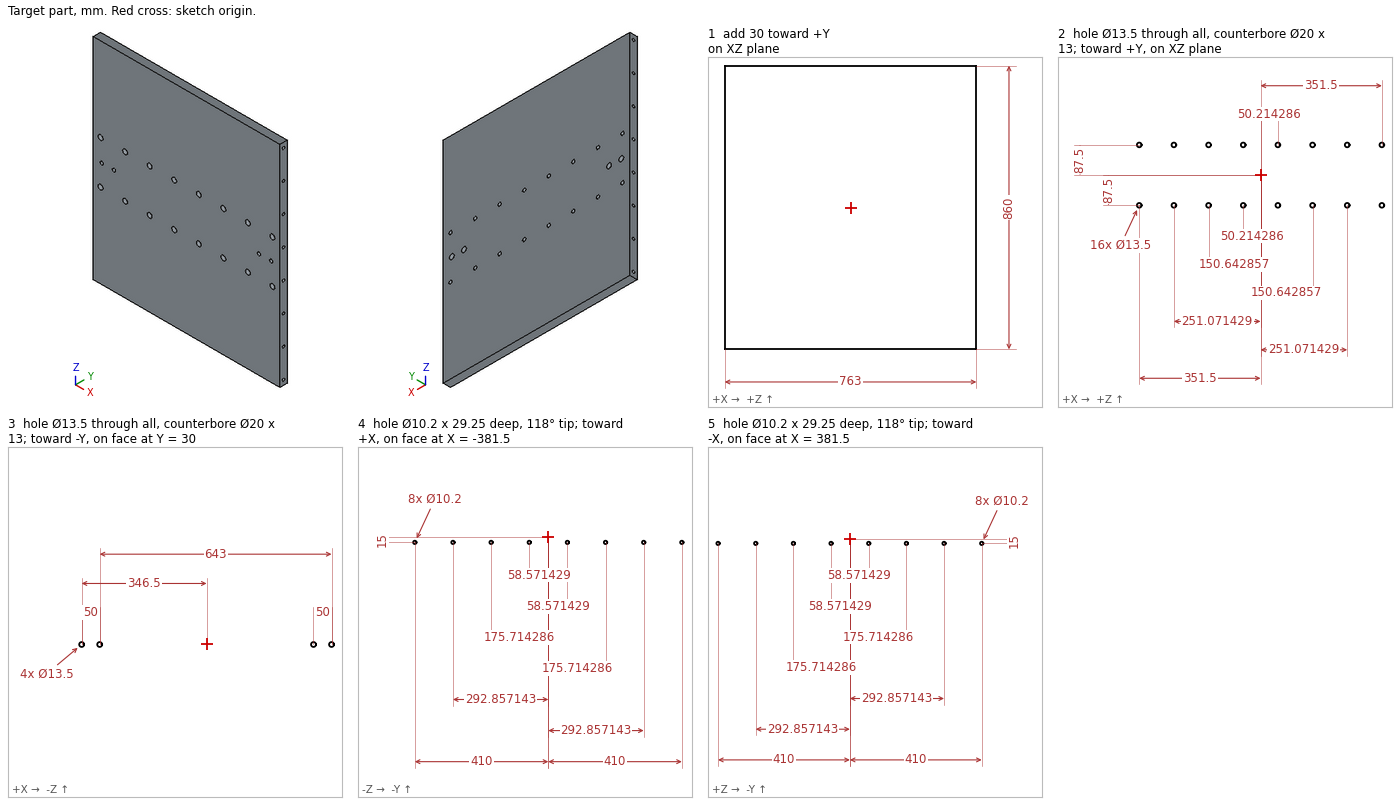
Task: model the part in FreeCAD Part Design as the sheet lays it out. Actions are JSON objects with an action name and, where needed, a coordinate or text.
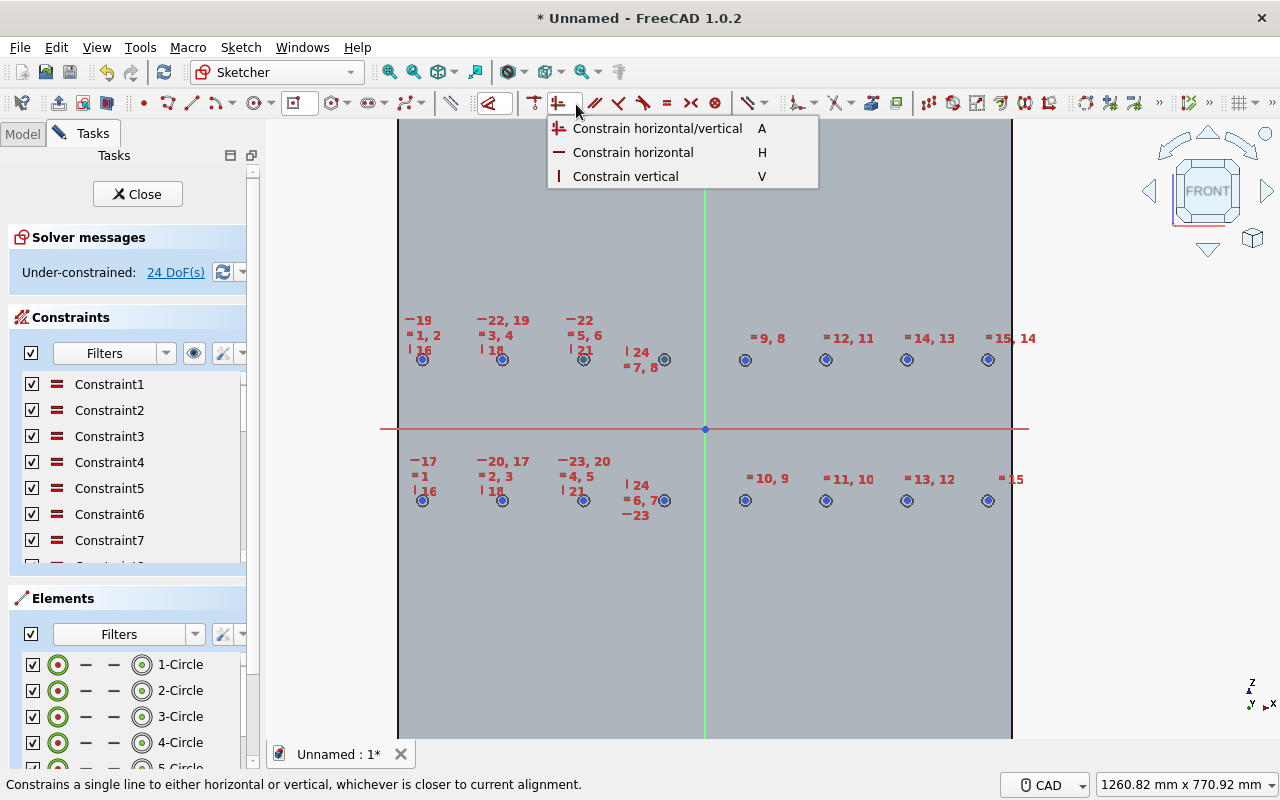
{"action": "left_click", "coordinate": [683, 152]}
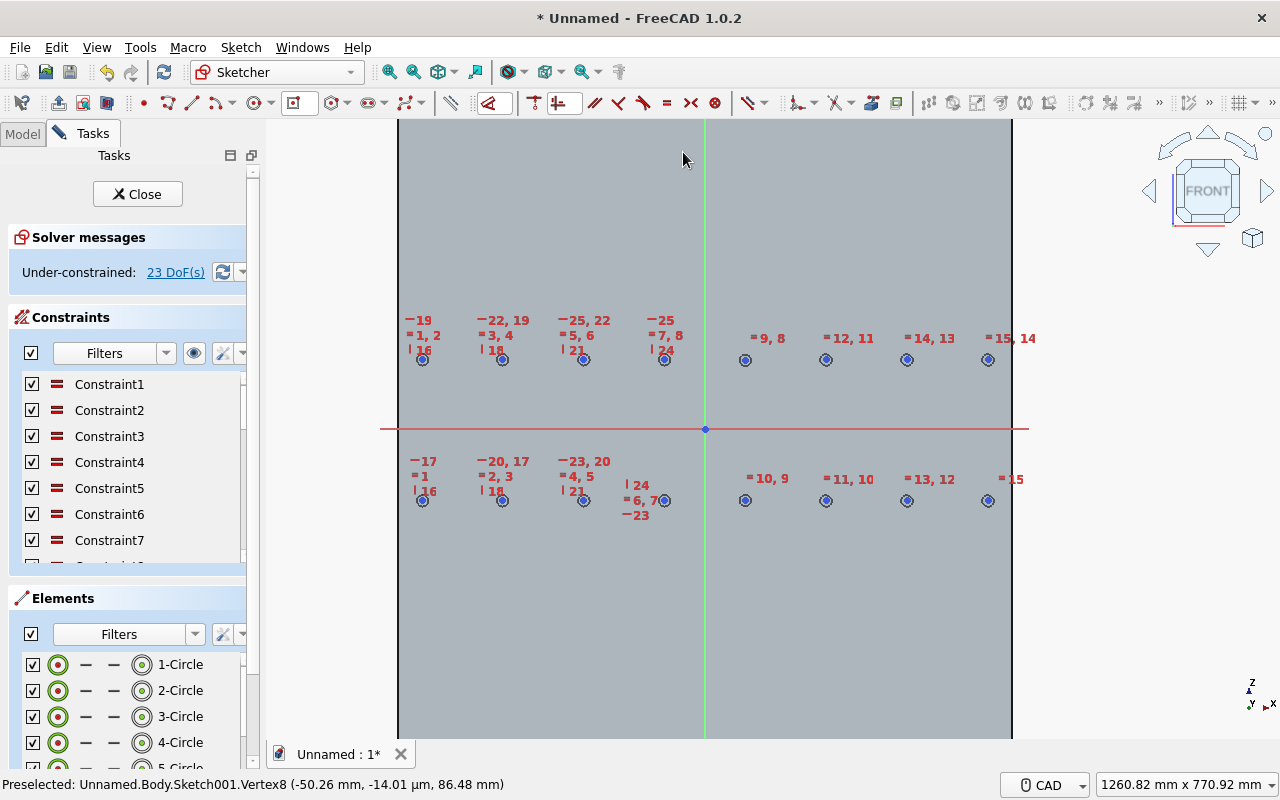
{"action": "left_click", "coordinate": [665, 360]}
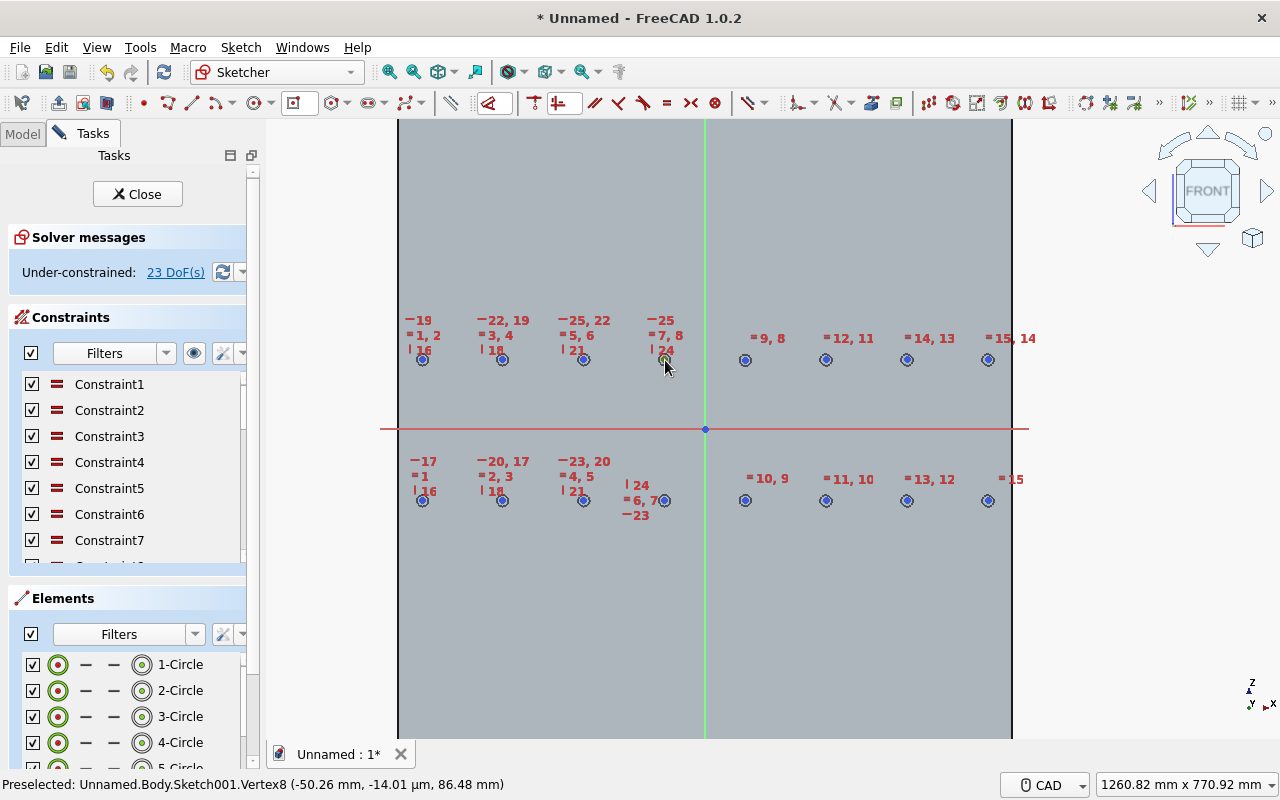
{"action": "left_click", "coordinate": [745, 360]}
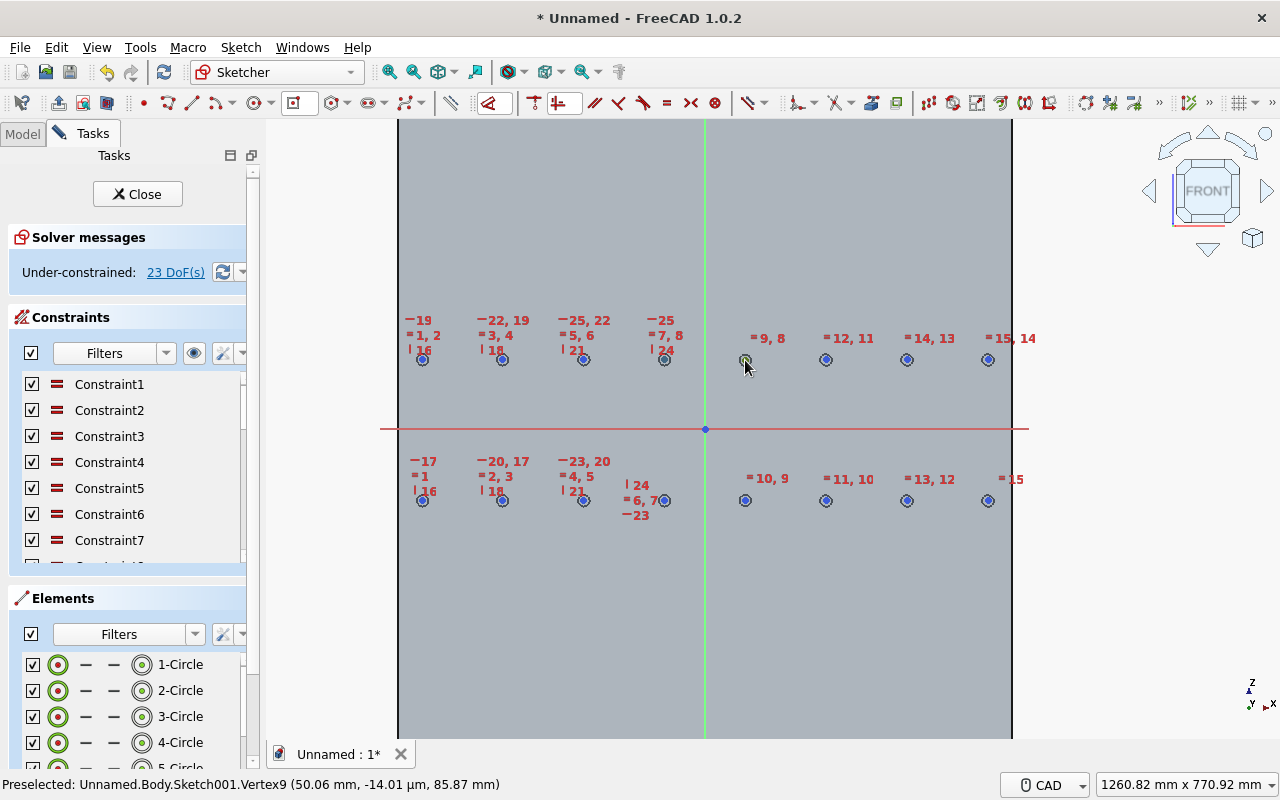
{"action": "key", "text": "h"}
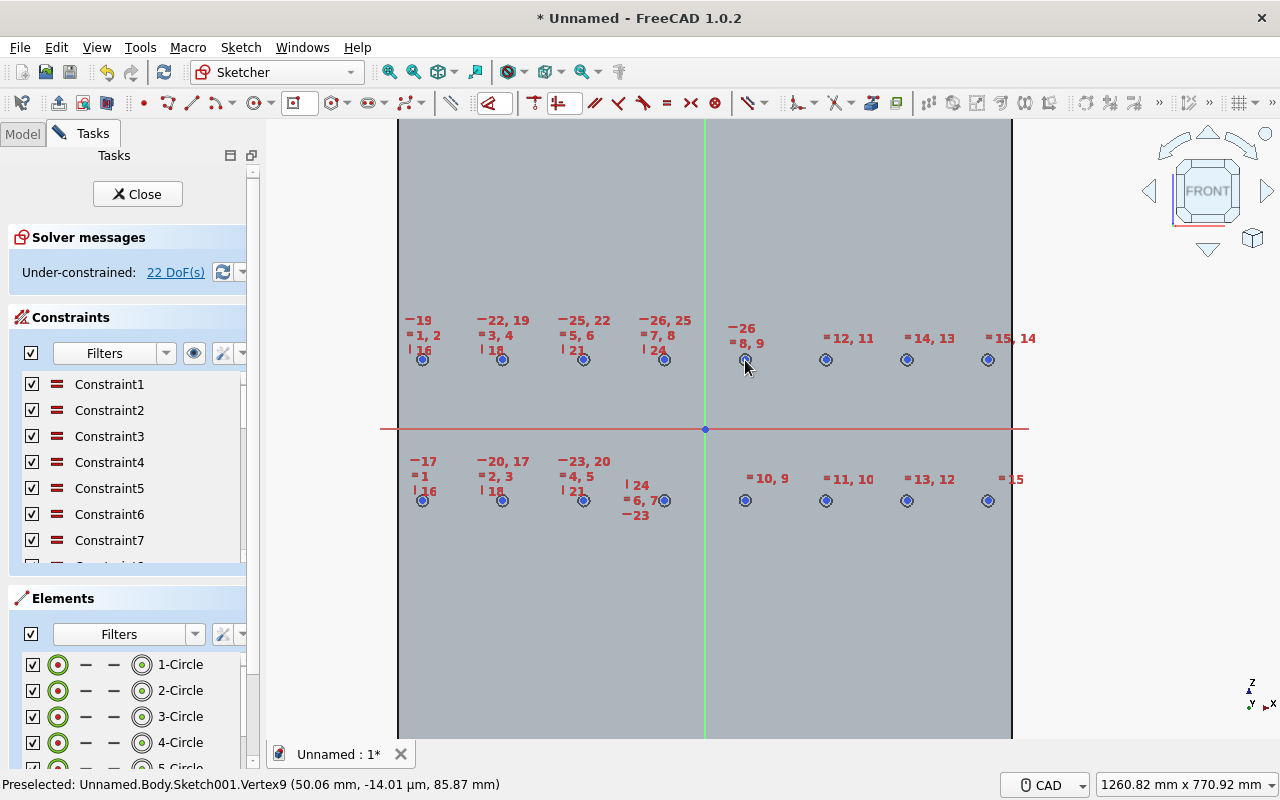
{"action": "left_click", "coordinate": [745, 360]}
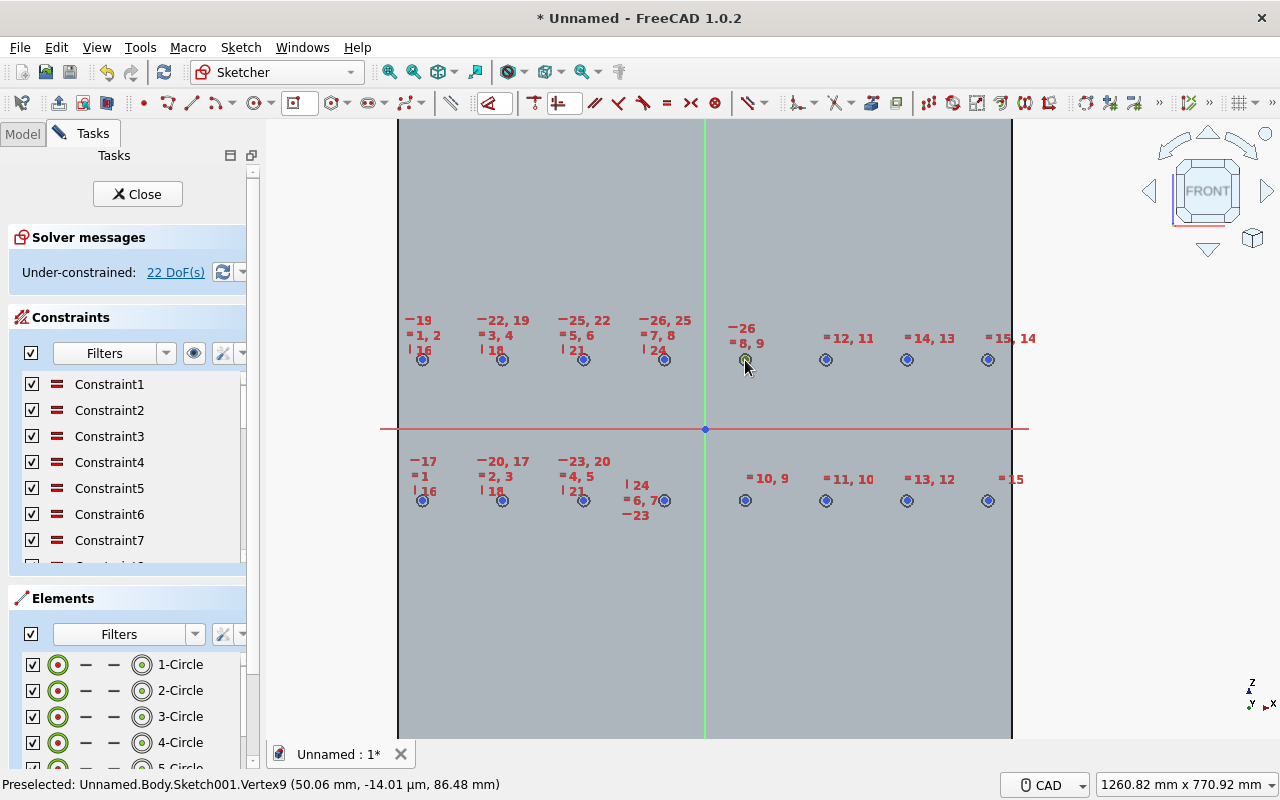
{"action": "left_click", "coordinate": [745, 501]}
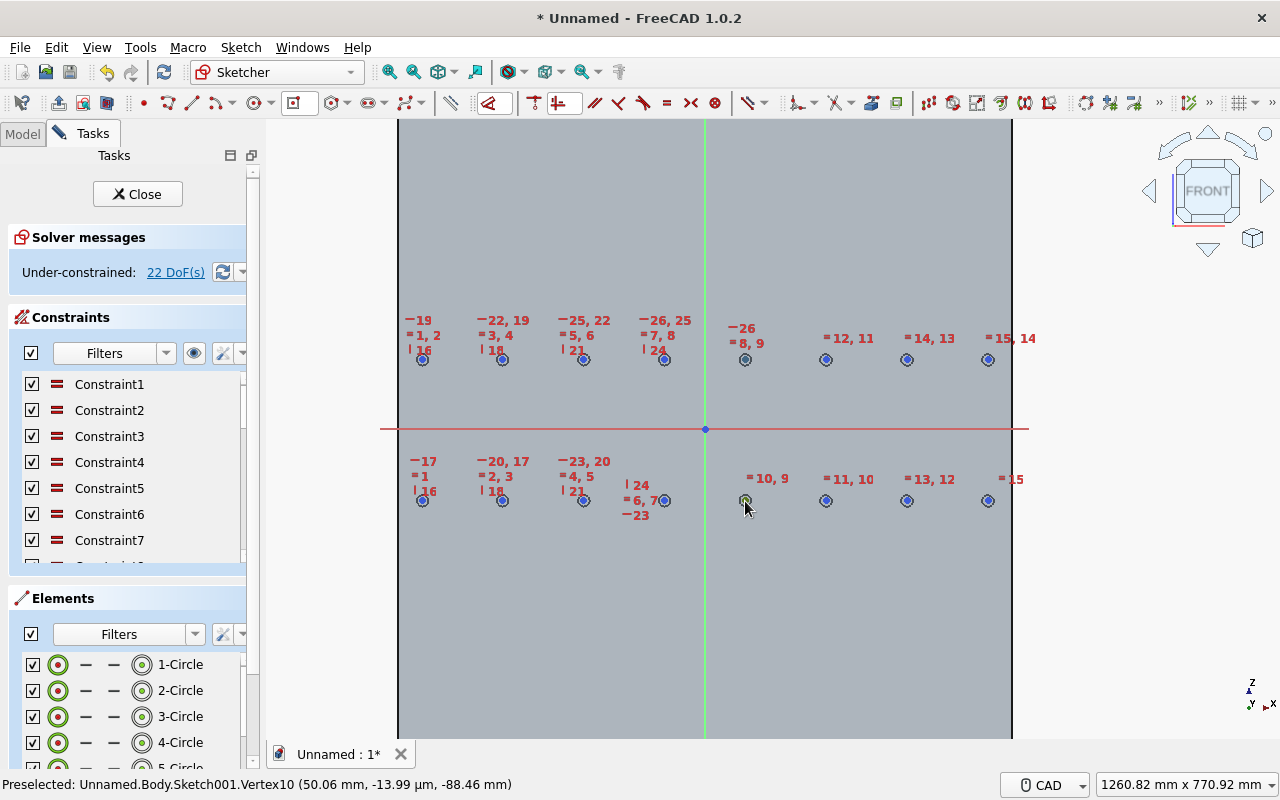
{"action": "left_click", "coordinate": [576, 104]}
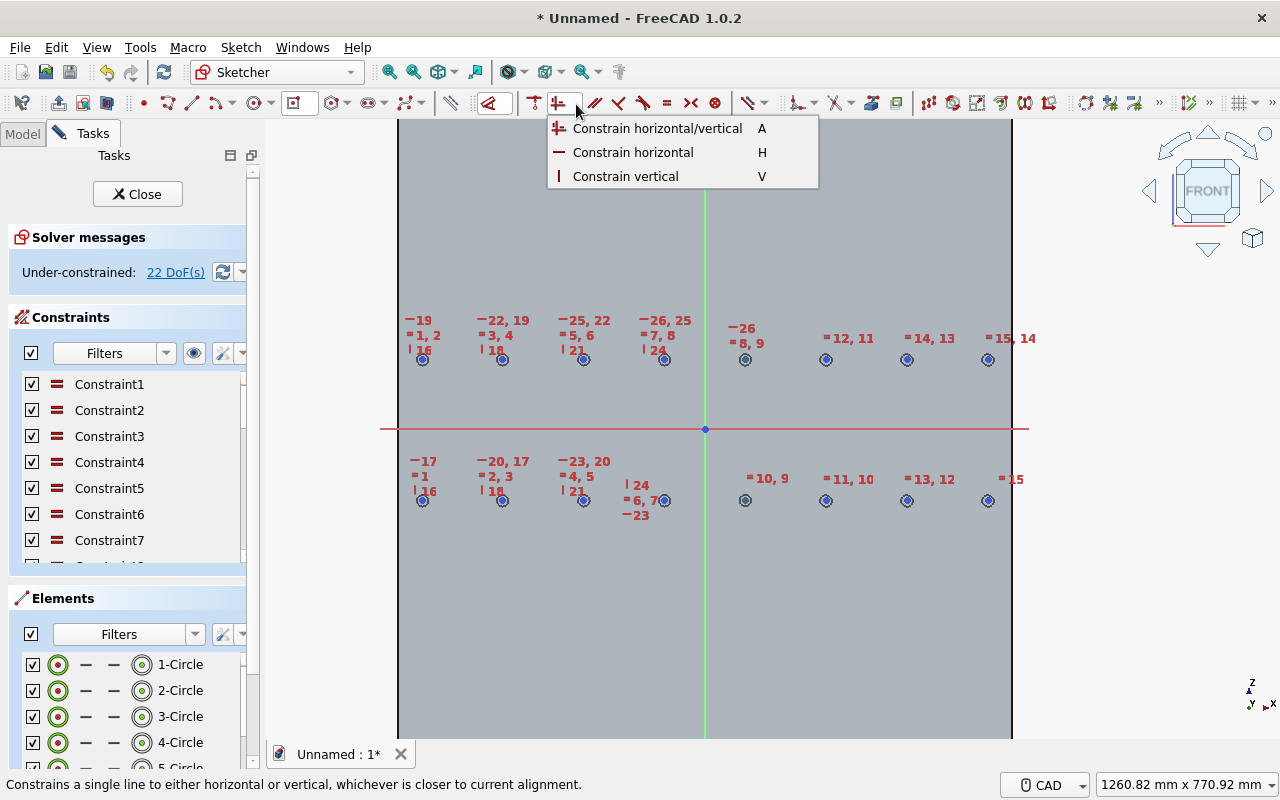
{"action": "left_click", "coordinate": [683, 176]}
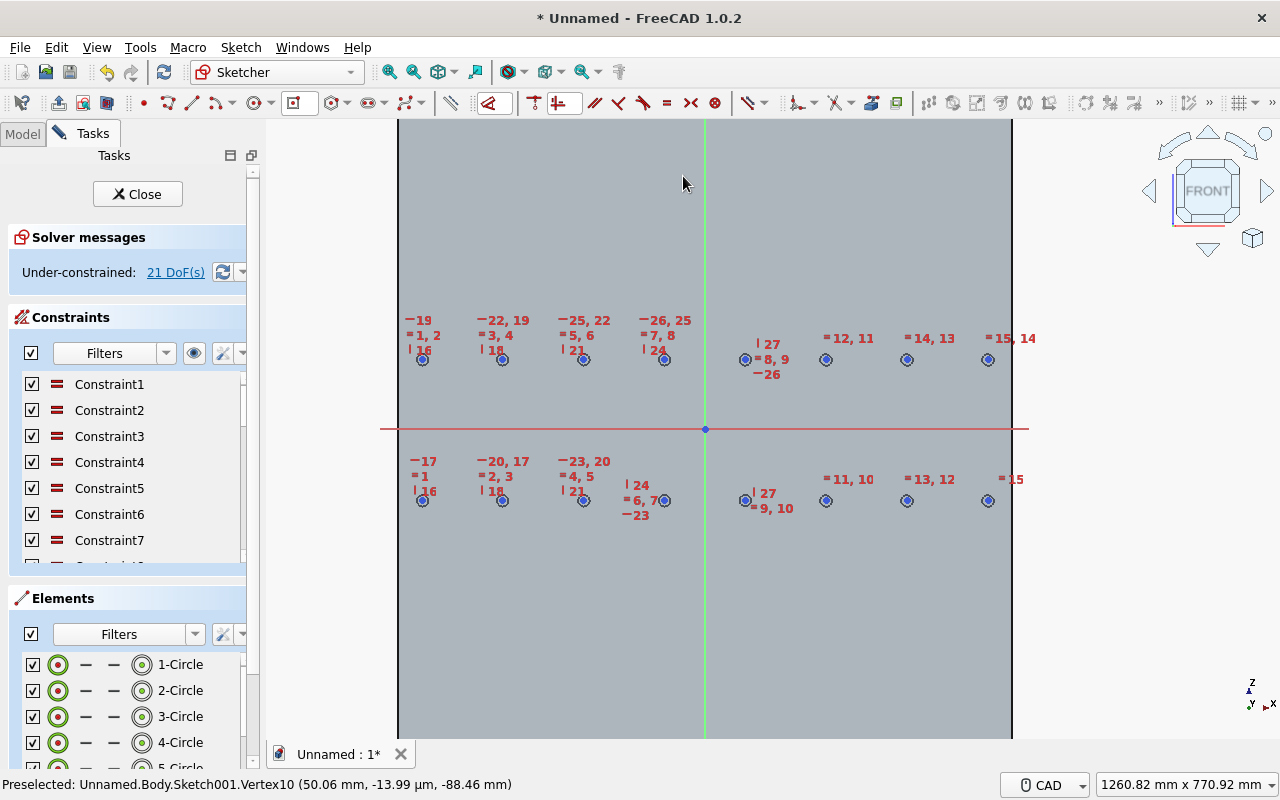
{"action": "left_click", "coordinate": [665, 501]}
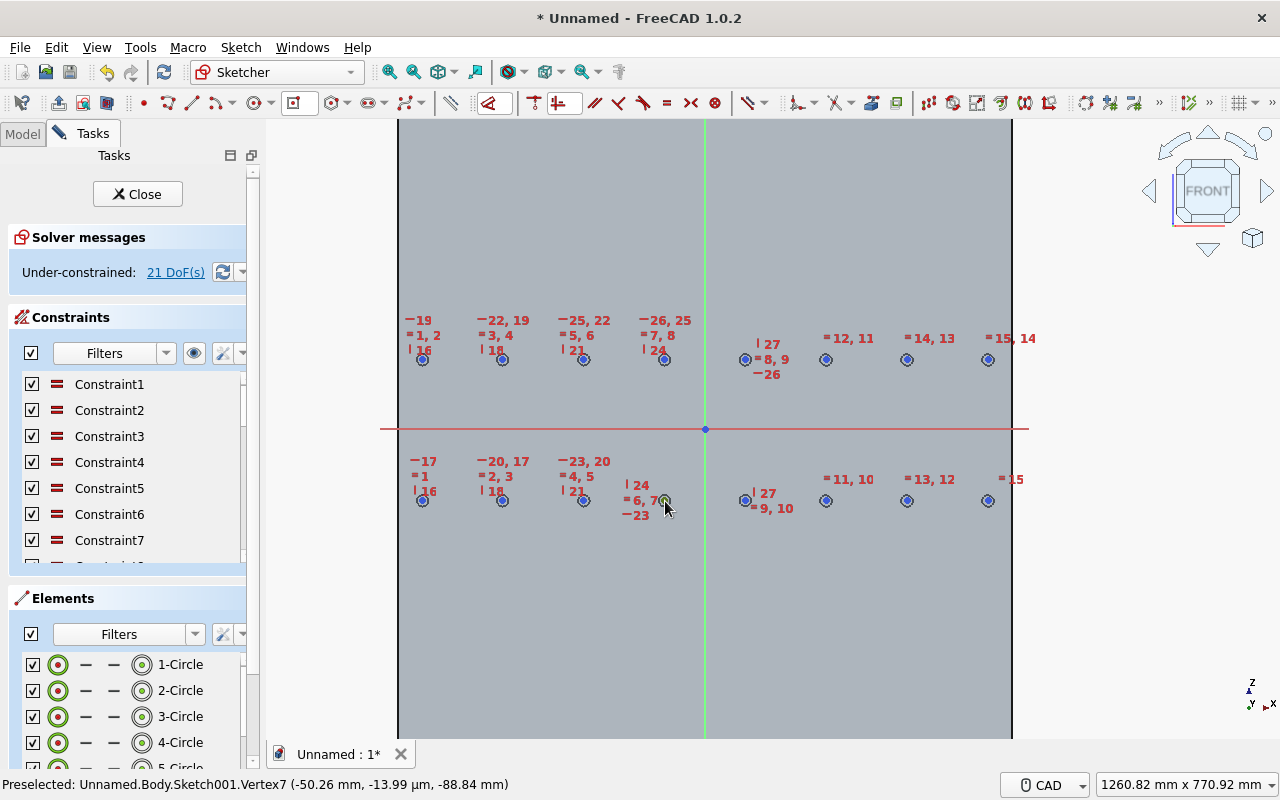
{"action": "left_click", "coordinate": [745, 501]}